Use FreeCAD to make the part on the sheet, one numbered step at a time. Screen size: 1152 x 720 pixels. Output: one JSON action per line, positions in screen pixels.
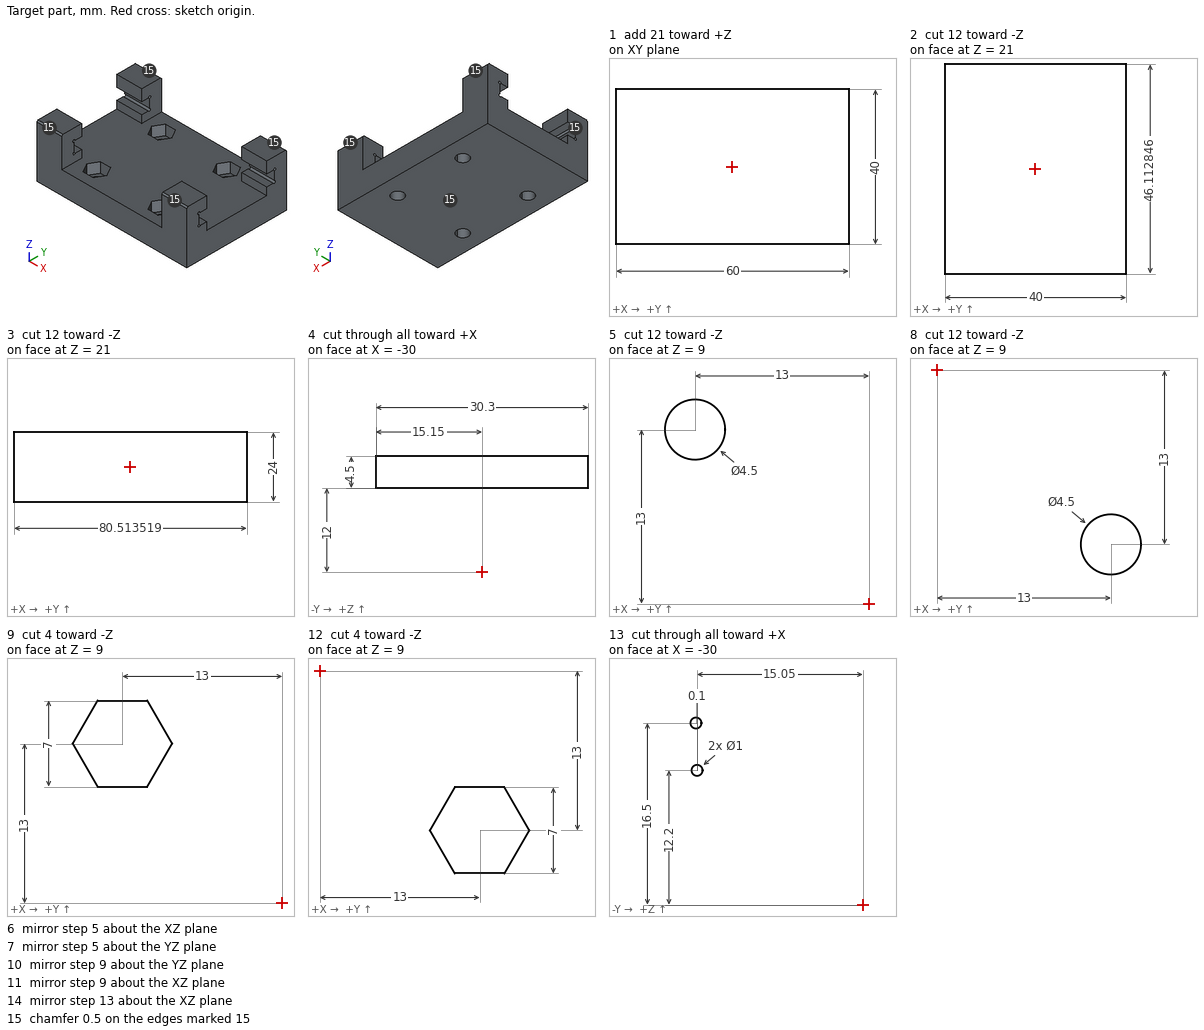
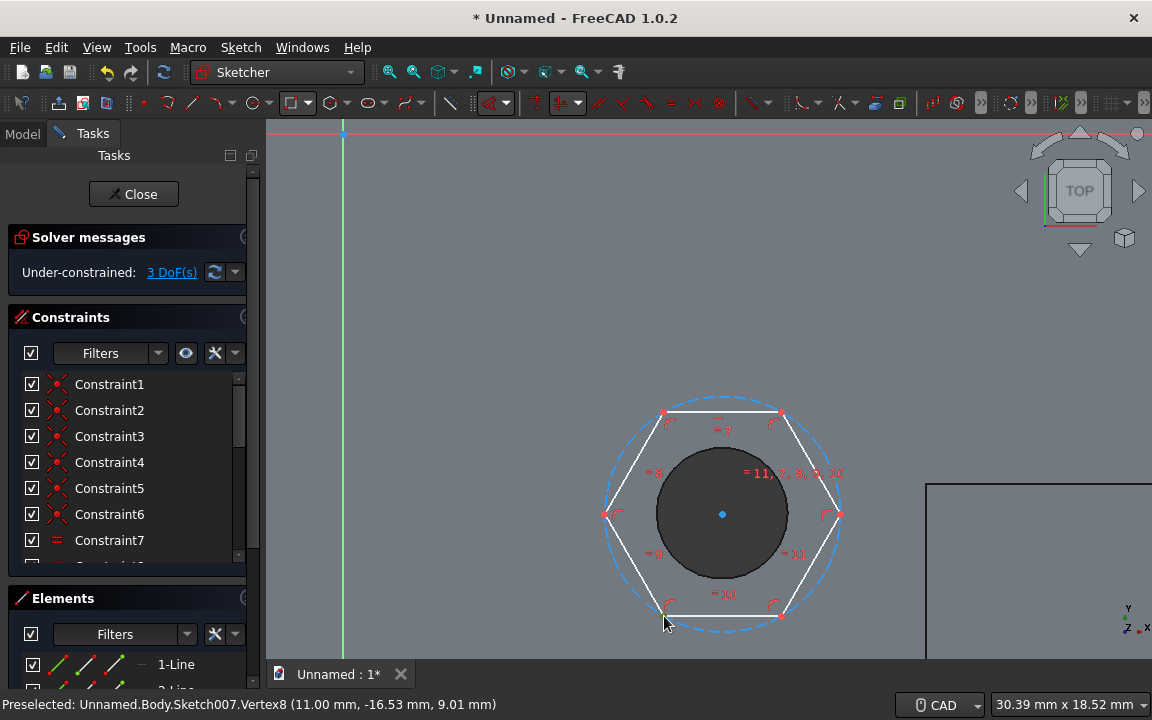
{"action": "left_click", "coordinate": [782, 412]}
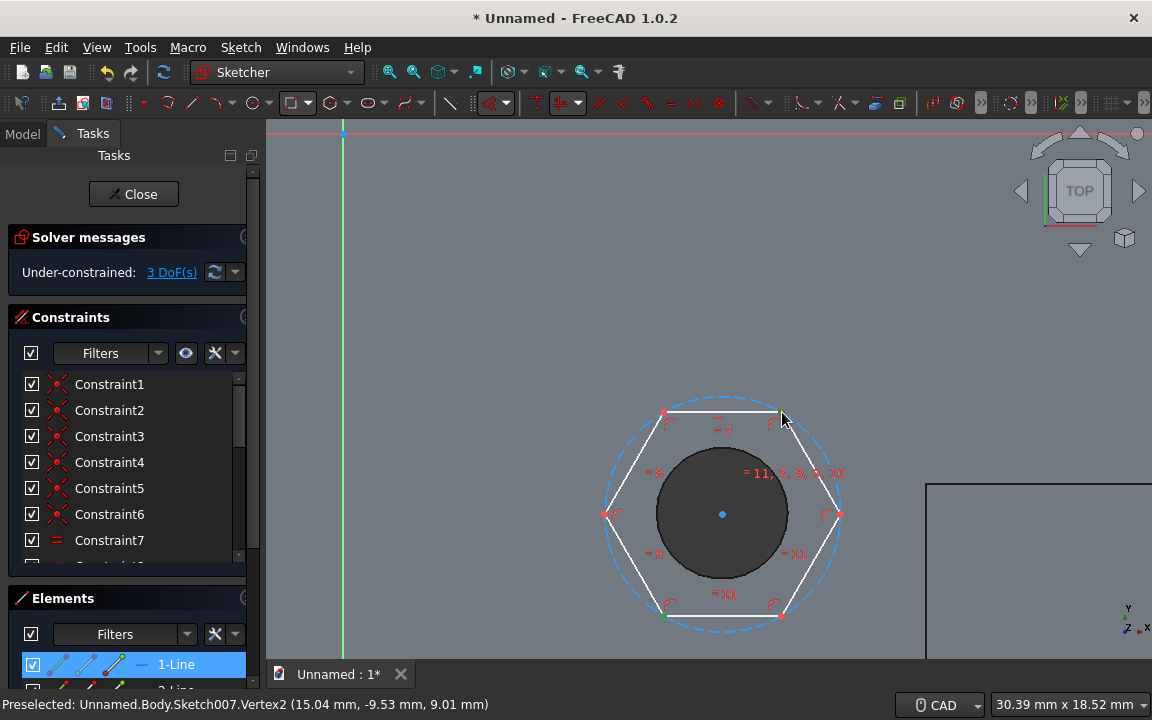
{"action": "key", "text": "i"}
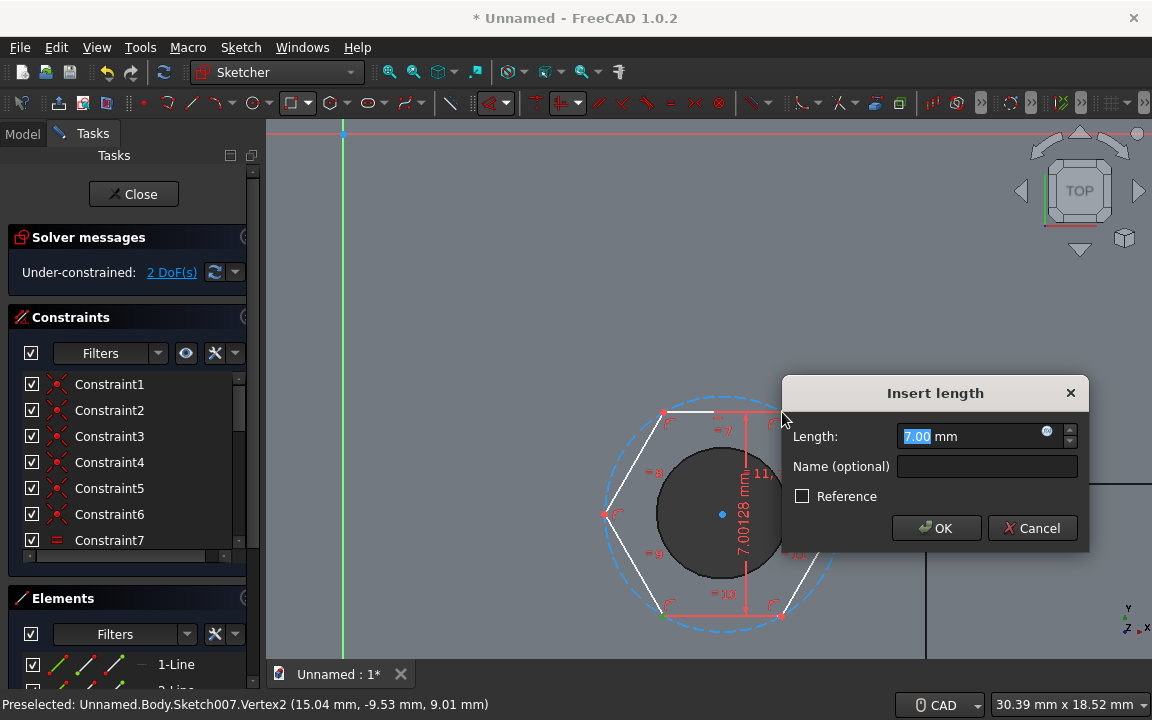
{"action": "type", "text": "7"}
{"action": "key", "text": "Return"}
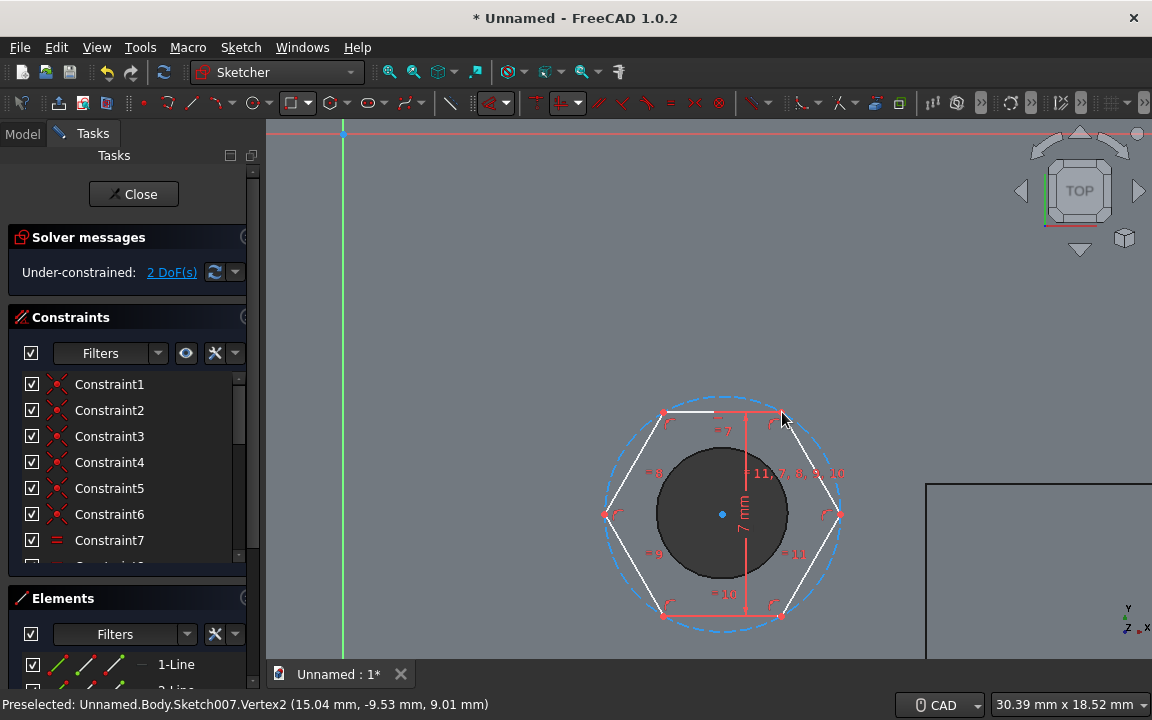
{"action": "left_click", "coordinate": [723, 514]}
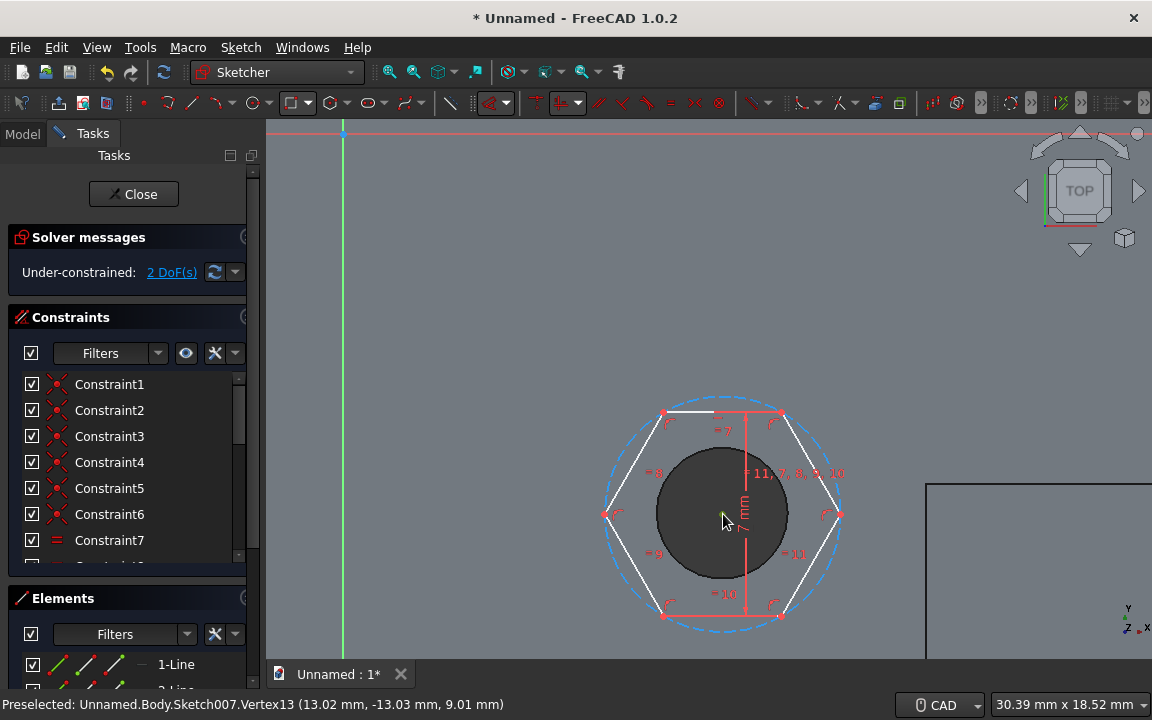
{"action": "left_click", "coordinate": [508, 104]}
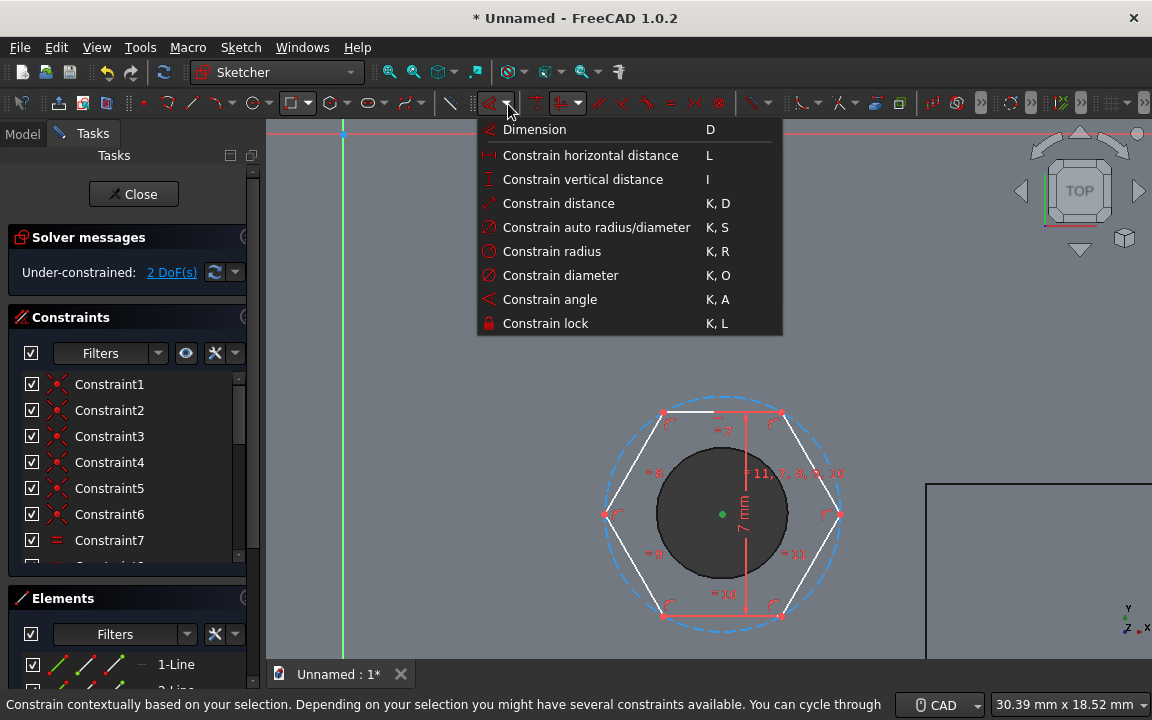
{"action": "left_click", "coordinate": [630, 155]}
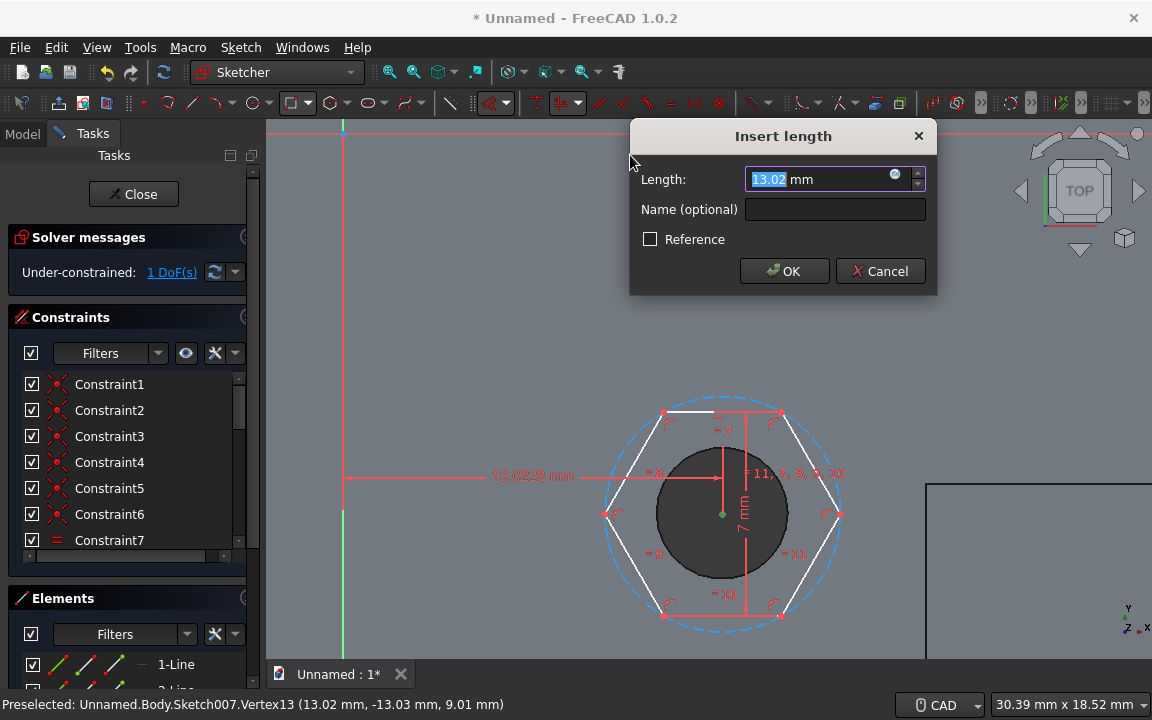
{"action": "type", "text": "13"}
{"action": "key", "text": "Return"}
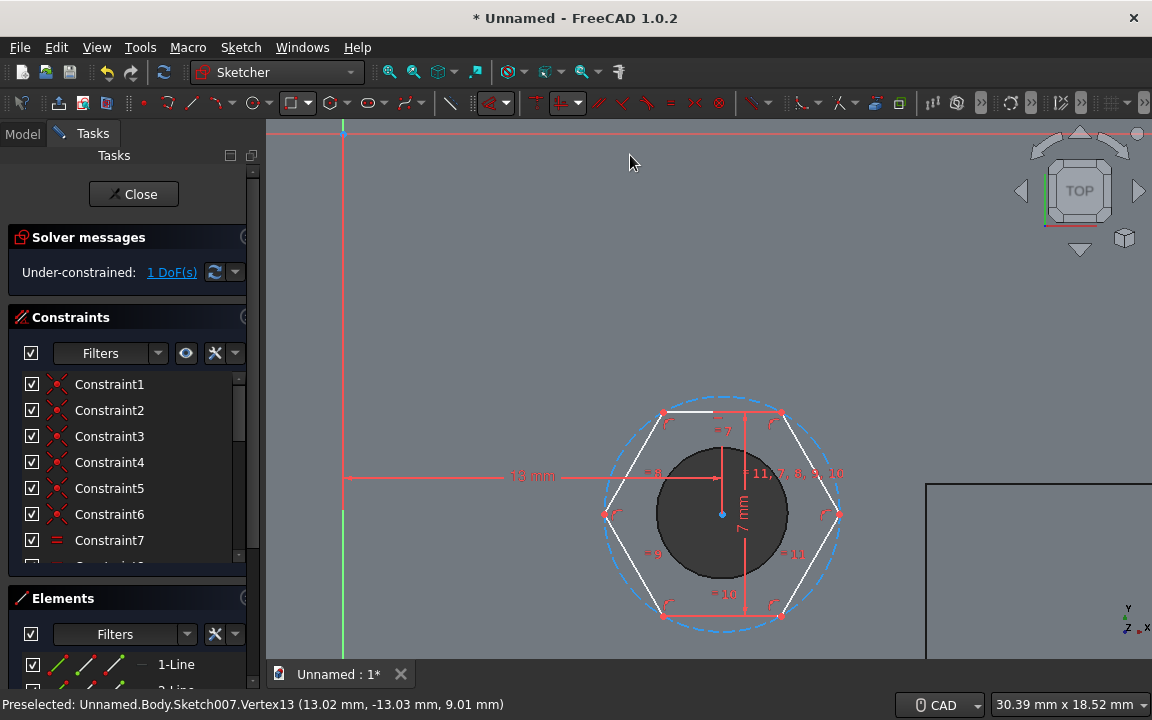
{"action": "left_click", "coordinate": [722, 514]}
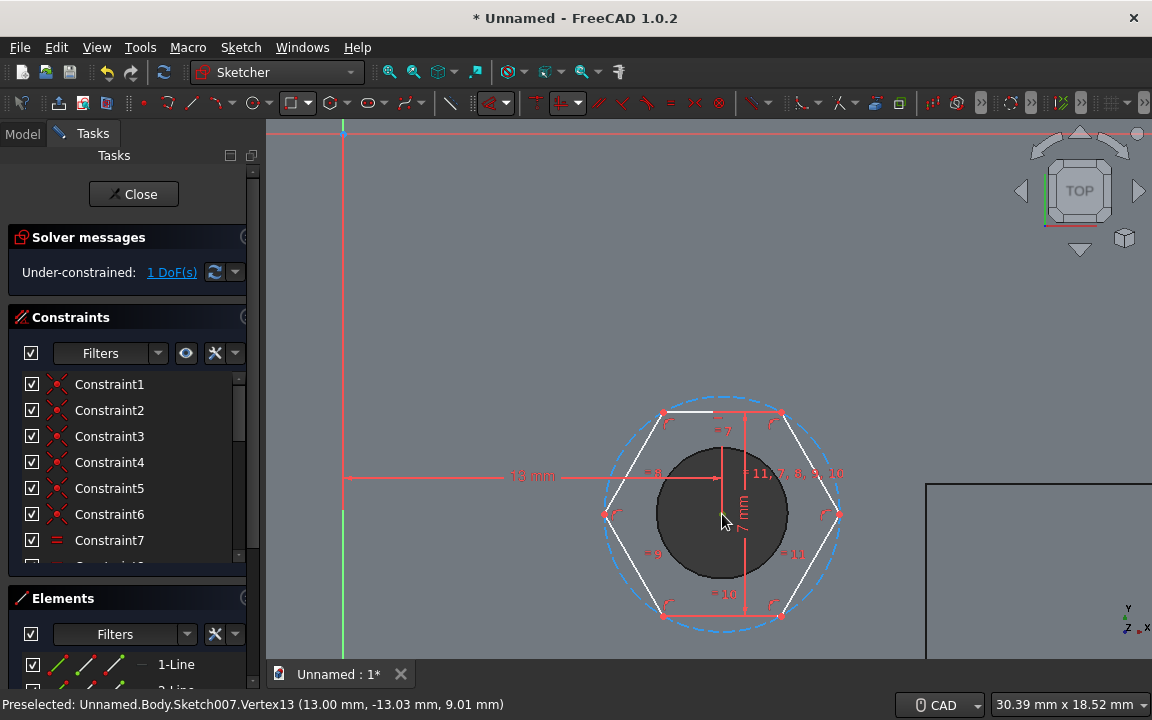
{"action": "left_click", "coordinate": [508, 104]}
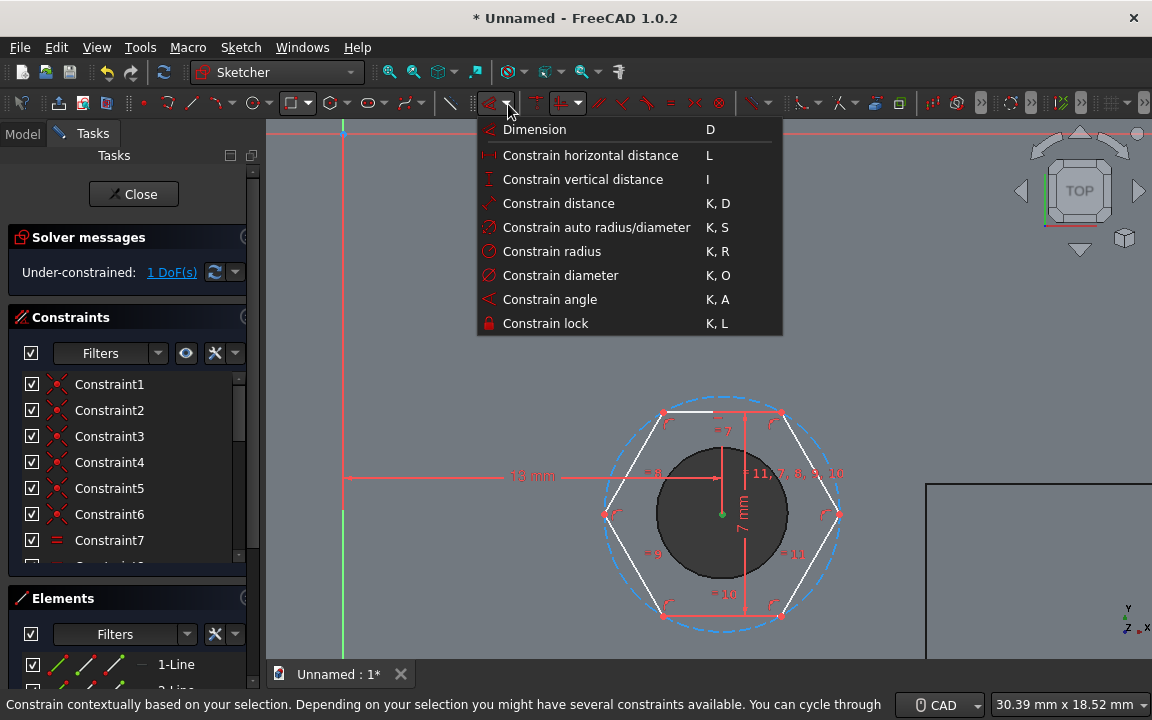
{"action": "left_click", "coordinate": [630, 179]}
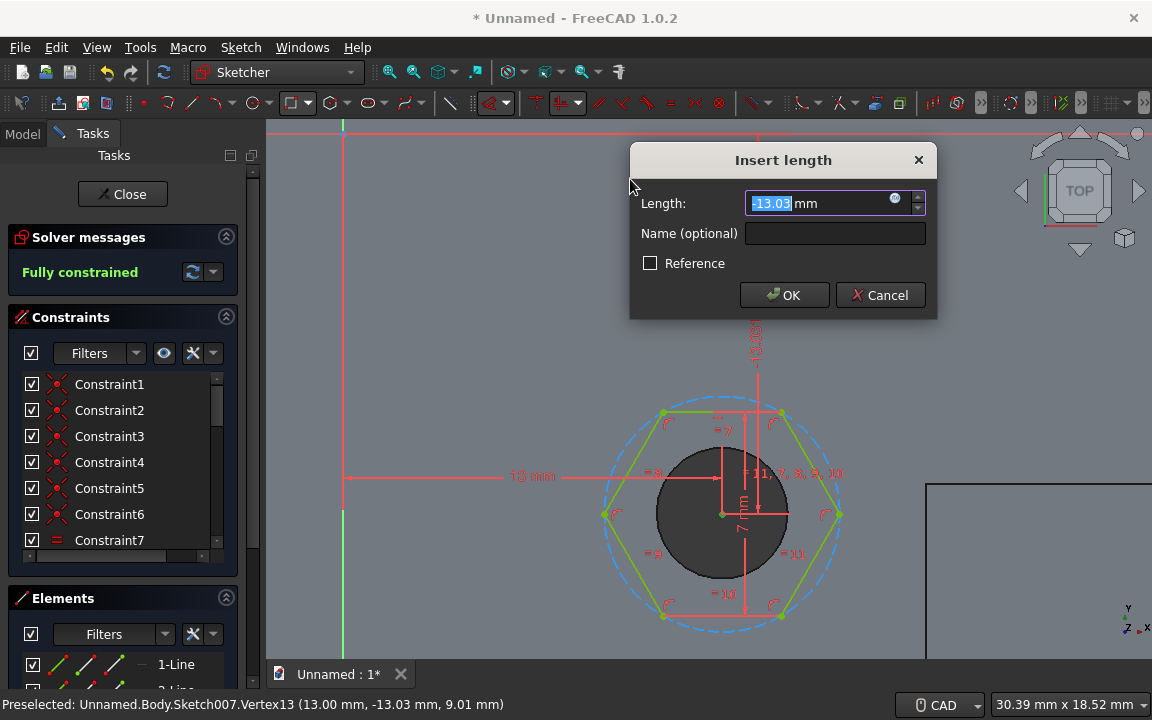
{"action": "type", "text": "-13"}
{"action": "key", "text": "Return"}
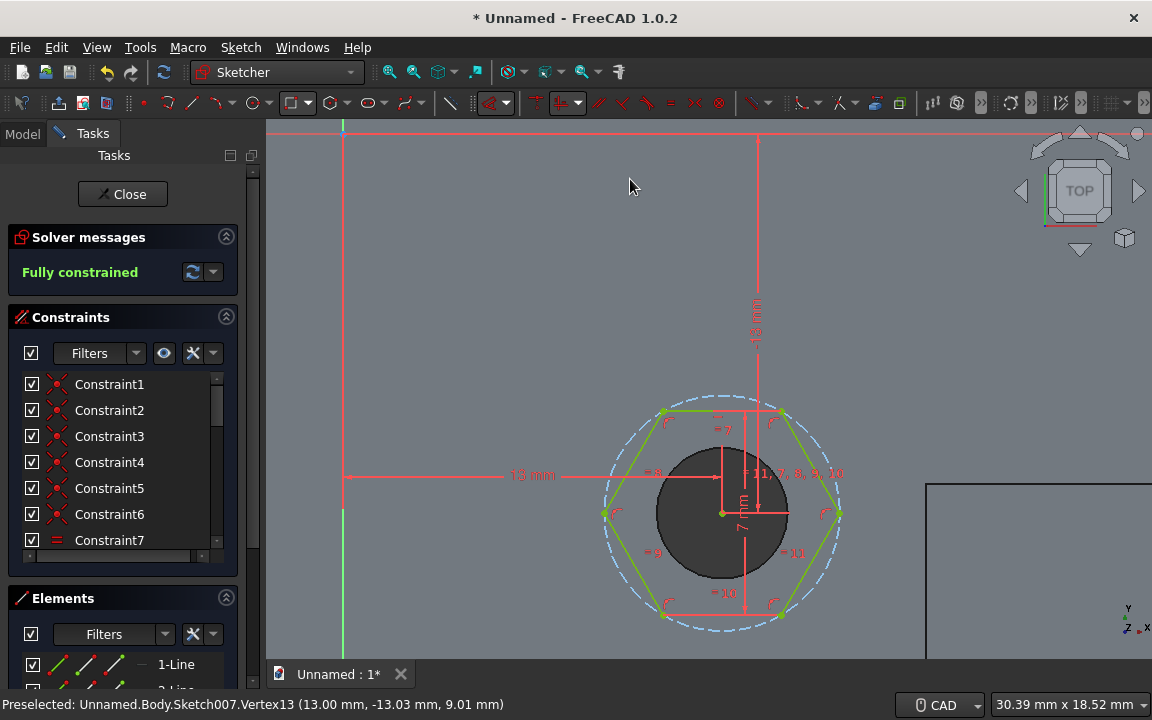
{"action": "left_click", "coordinate": [123, 194]}